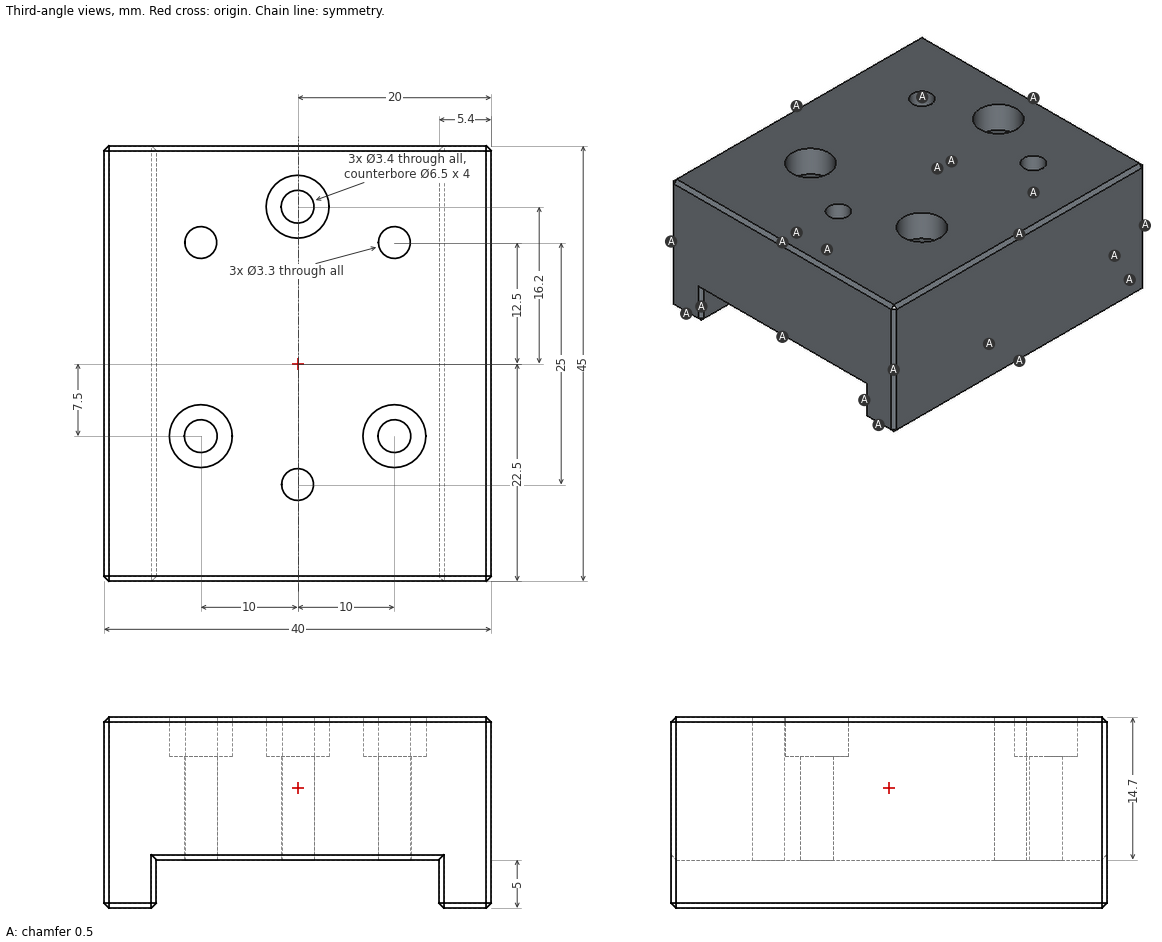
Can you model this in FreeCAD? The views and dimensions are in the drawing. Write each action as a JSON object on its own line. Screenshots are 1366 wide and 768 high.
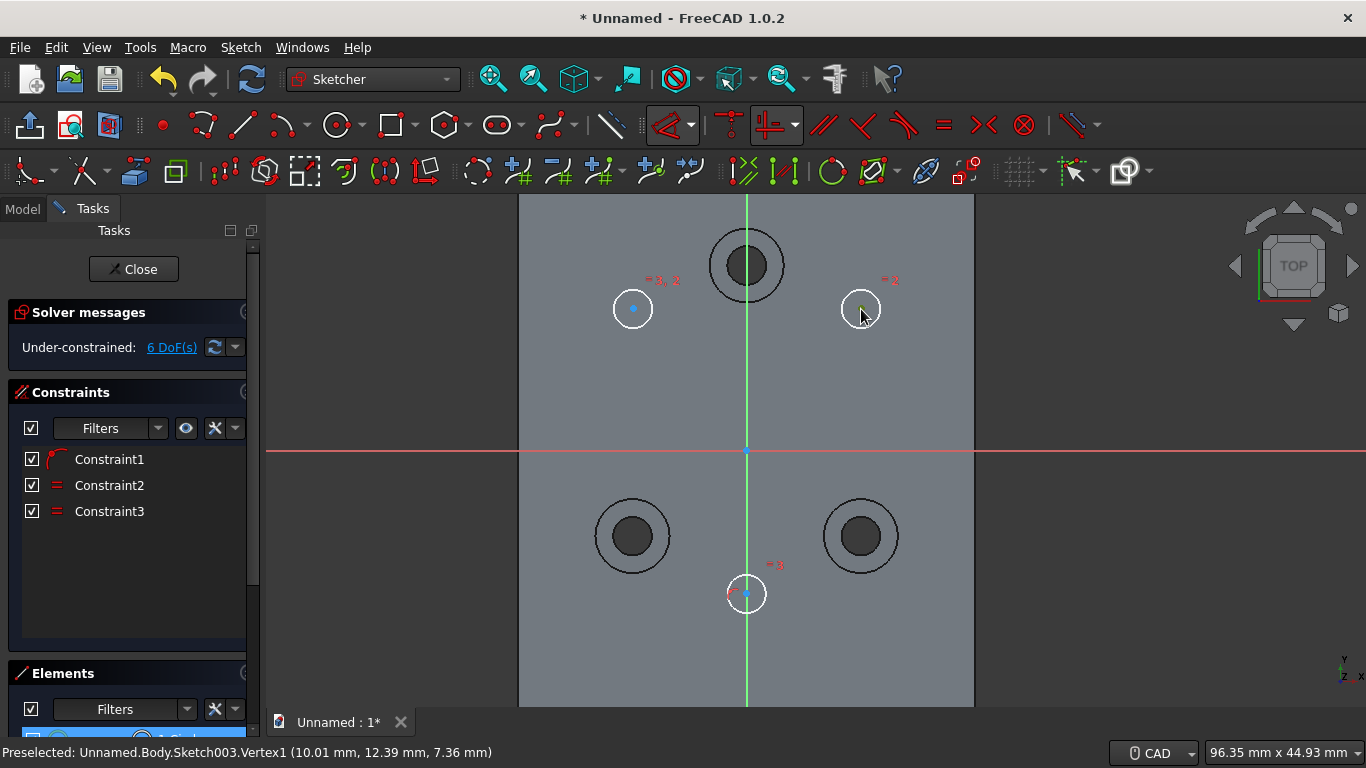
{"action": "left_click", "coordinate": [633, 309]}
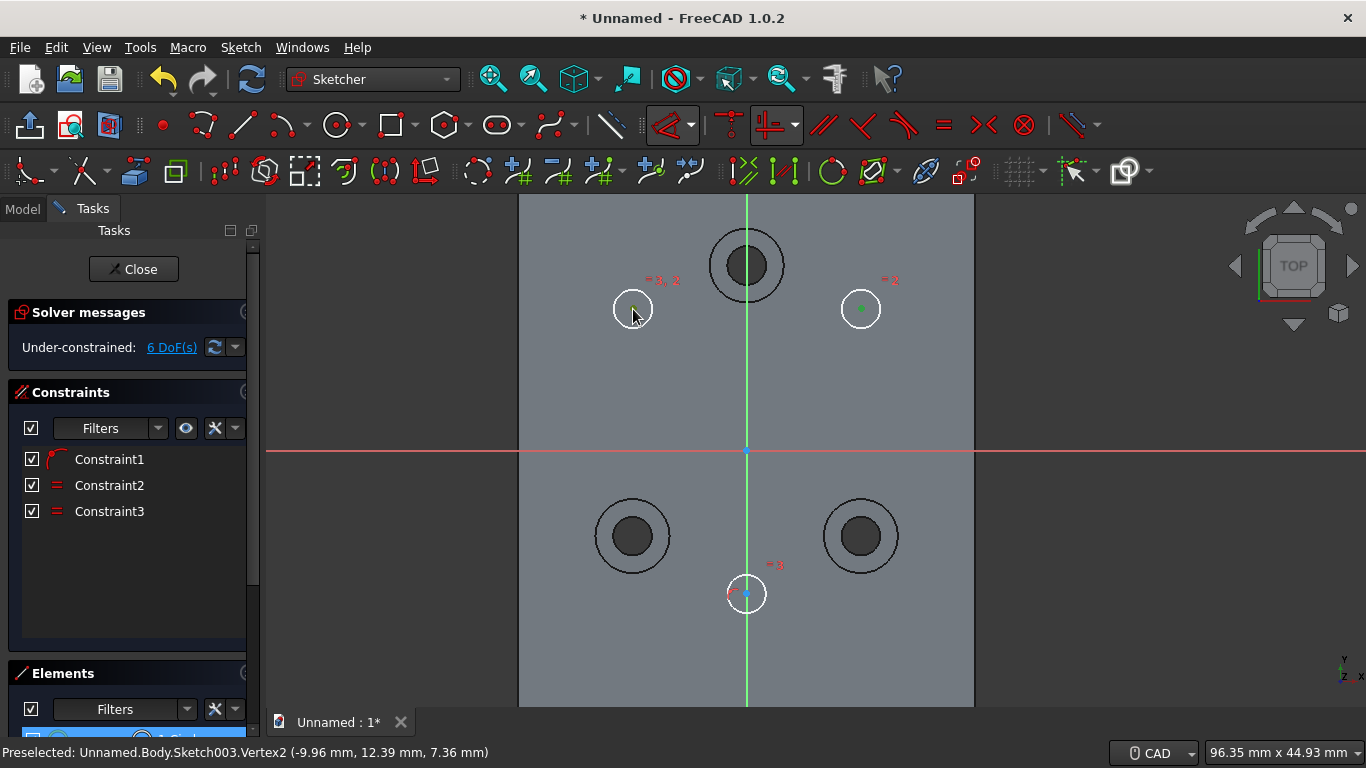
{"action": "key", "text": "h"}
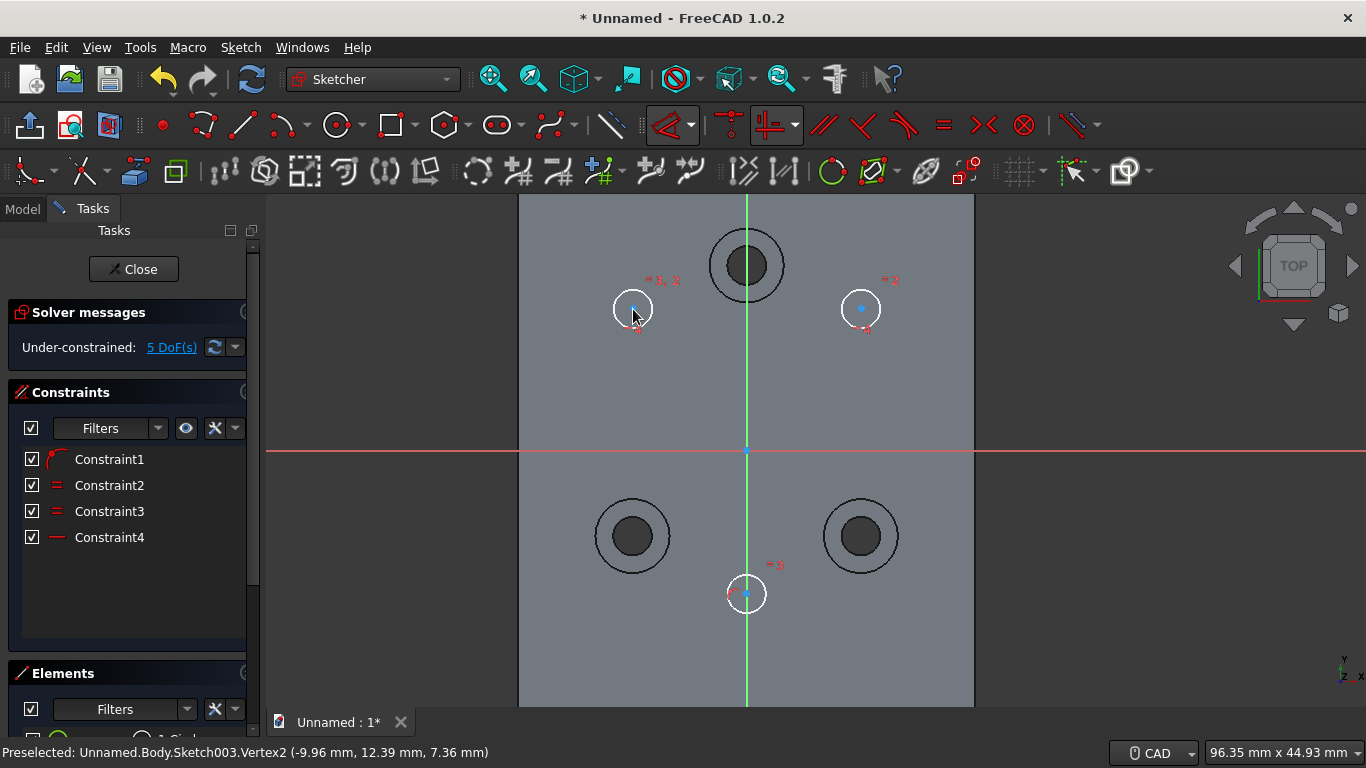
{"action": "left_click", "coordinate": [874, 295]}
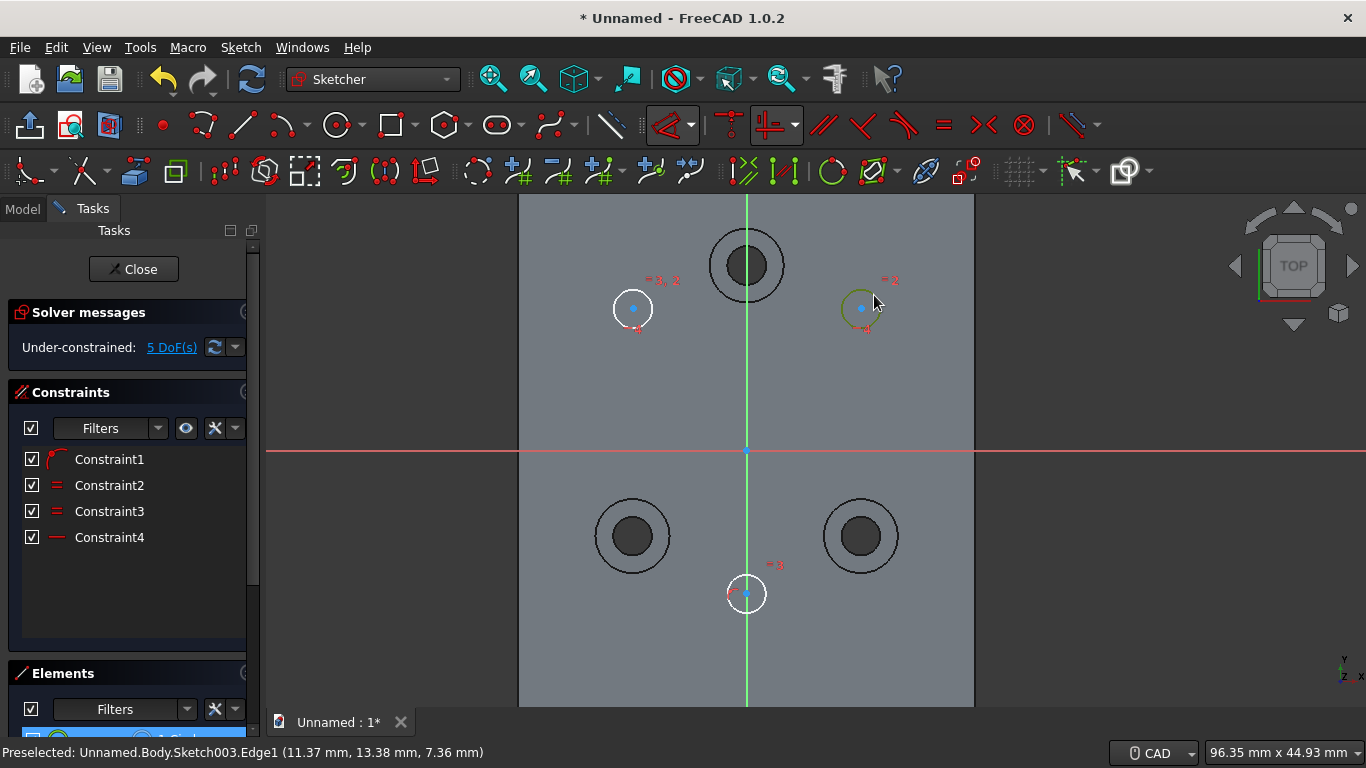
{"action": "left_click", "coordinate": [694, 126]}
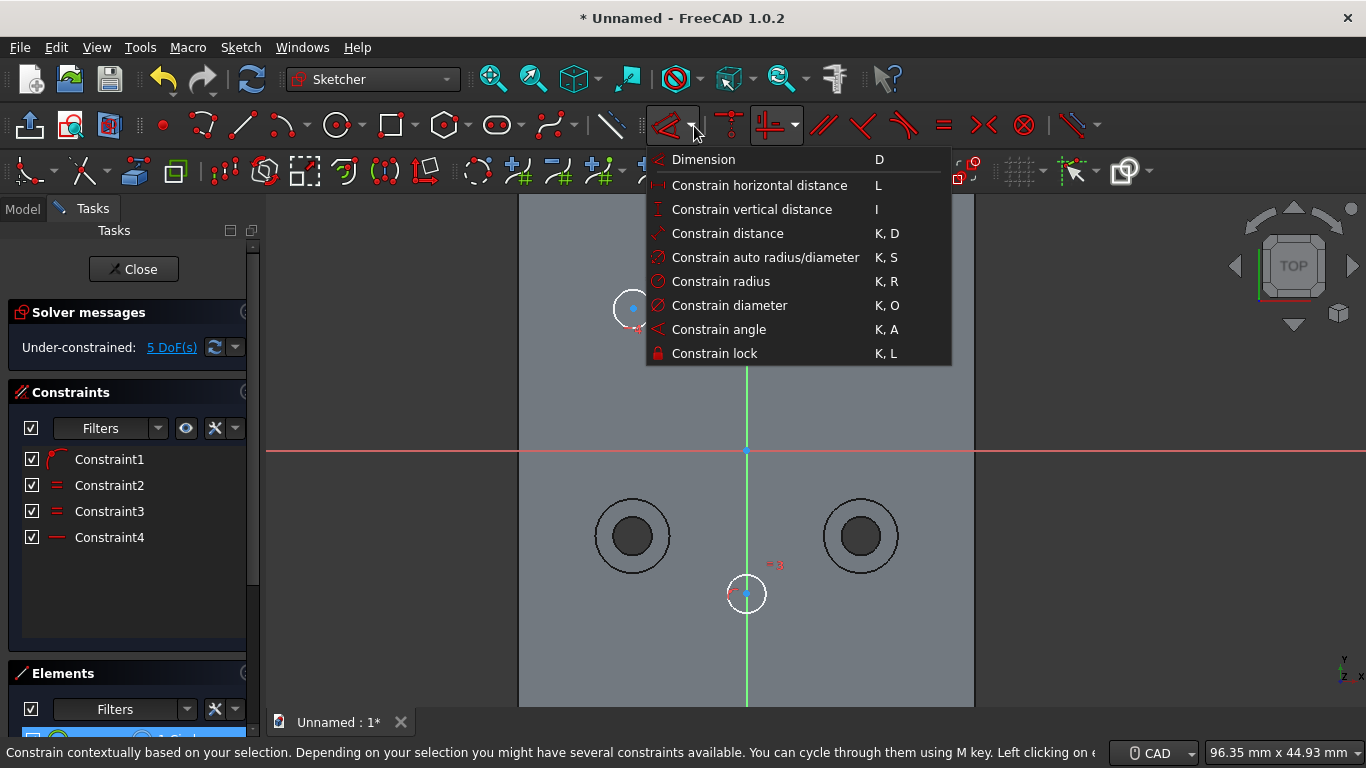
{"action": "left_click", "coordinate": [799, 305]}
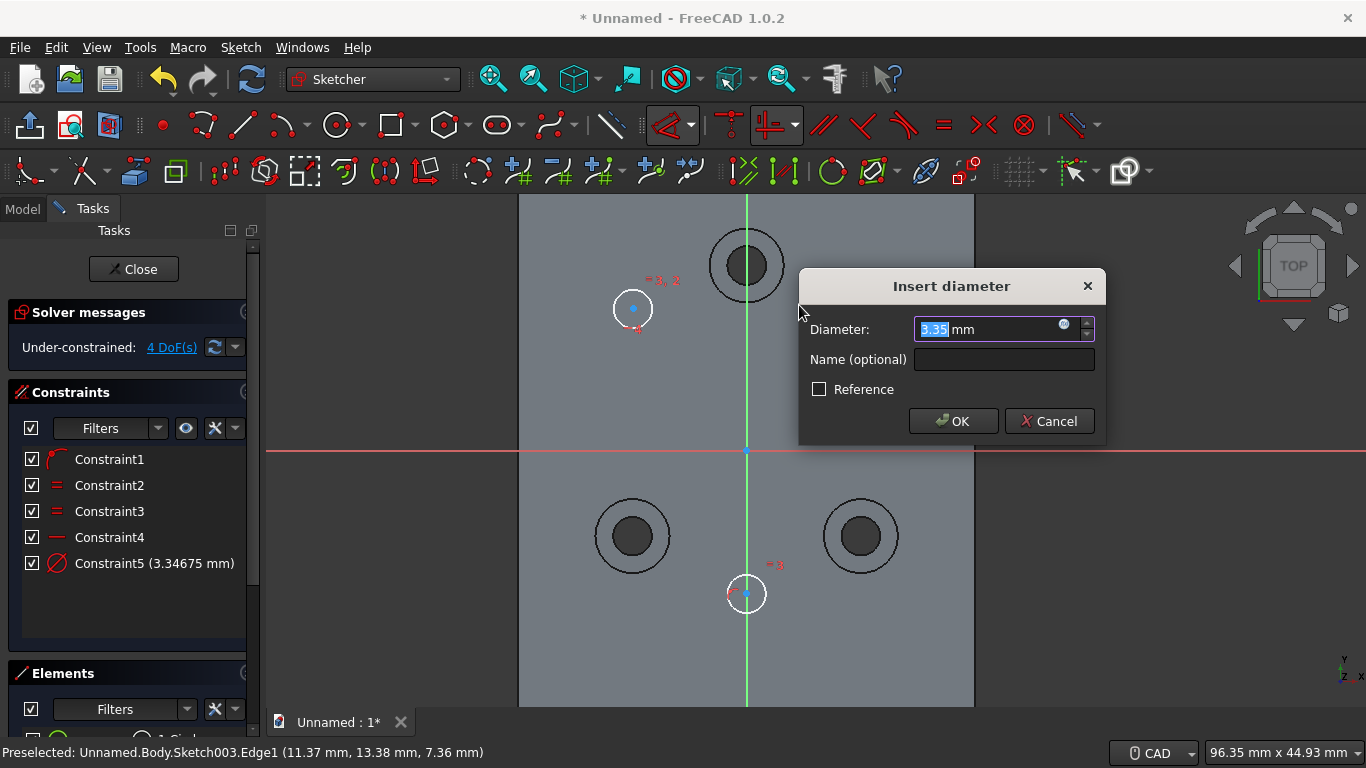
{"action": "type", "text": "3.3"}
{"action": "key", "text": "Return"}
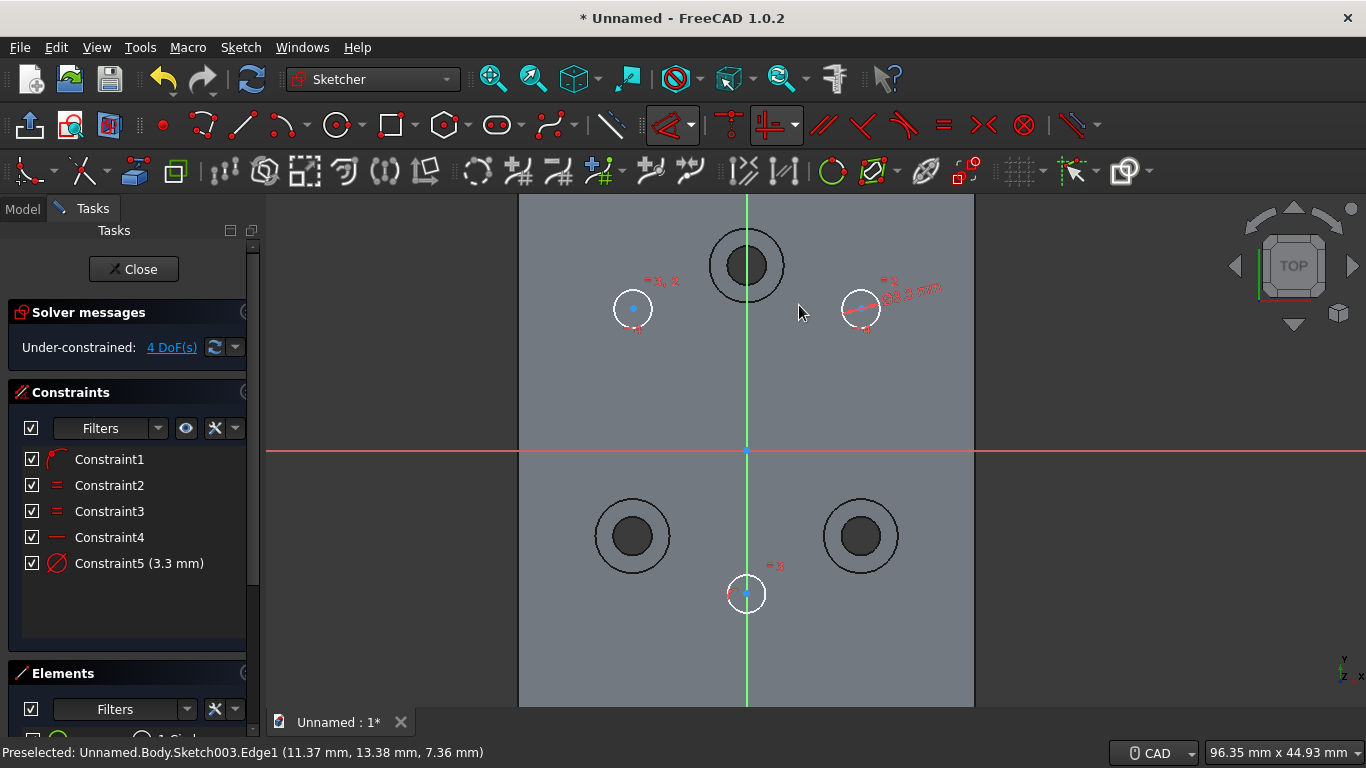
{"action": "left_click", "coordinate": [861, 309]}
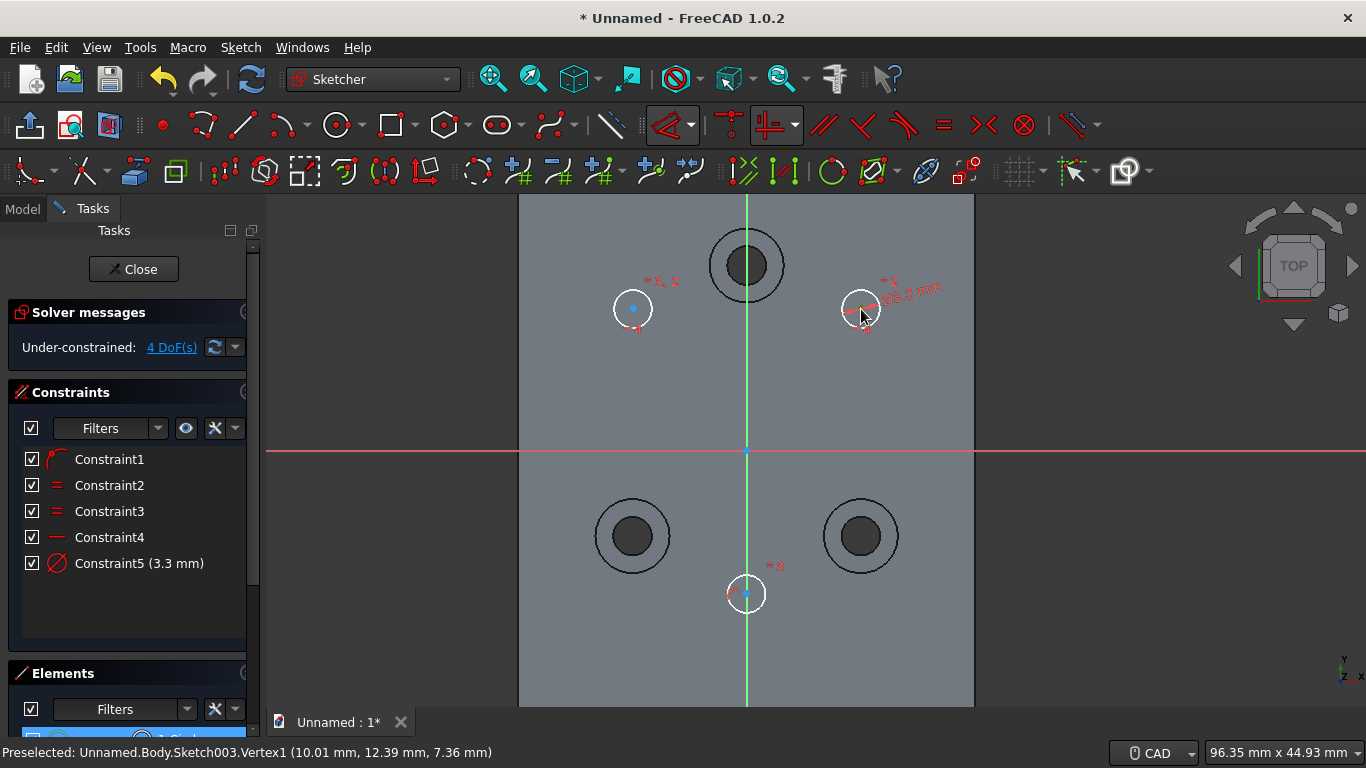
{"action": "key", "text": "l"}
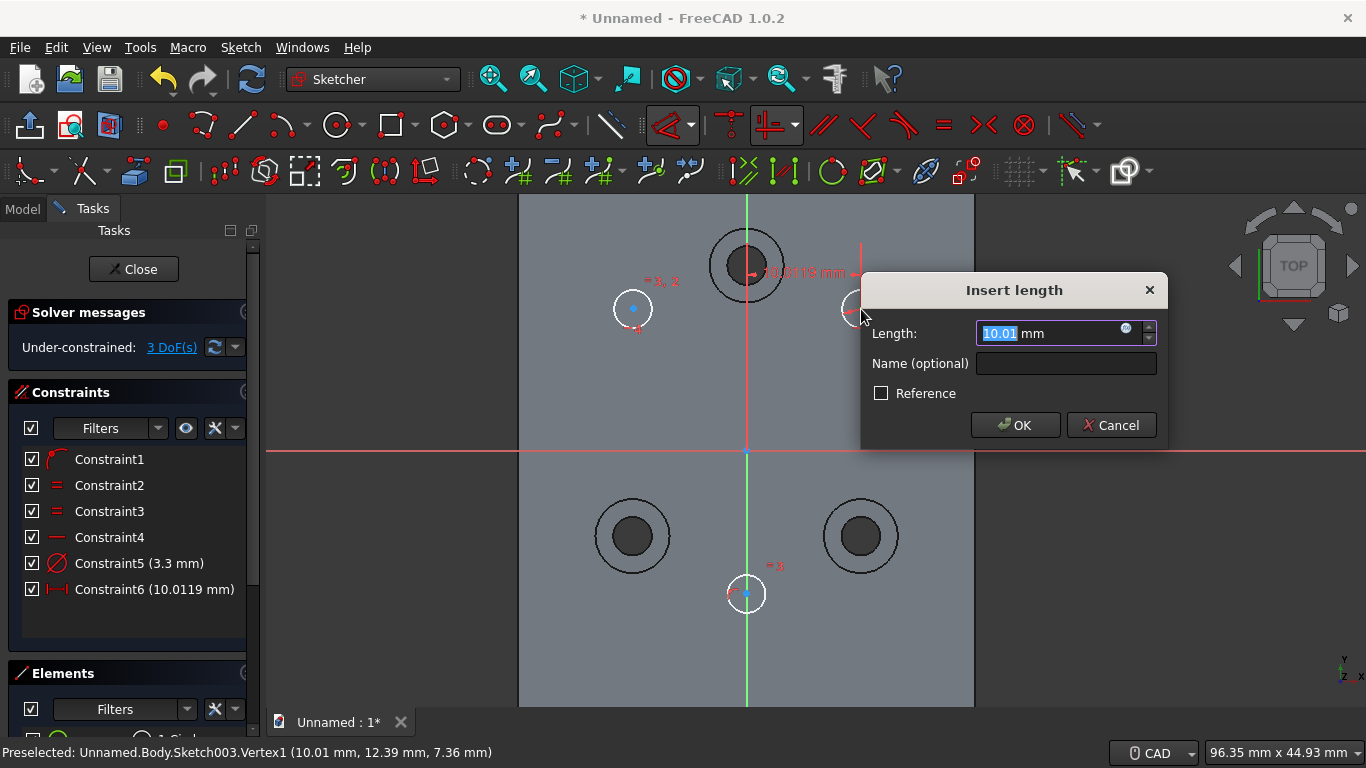
{"action": "type", "text": "10"}
{"action": "key", "text": "Return"}